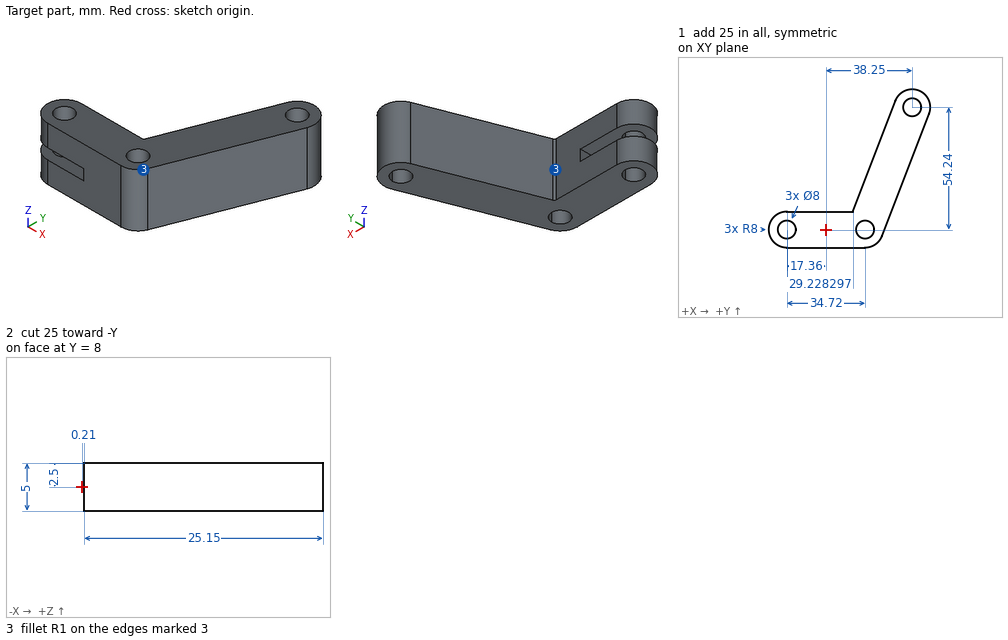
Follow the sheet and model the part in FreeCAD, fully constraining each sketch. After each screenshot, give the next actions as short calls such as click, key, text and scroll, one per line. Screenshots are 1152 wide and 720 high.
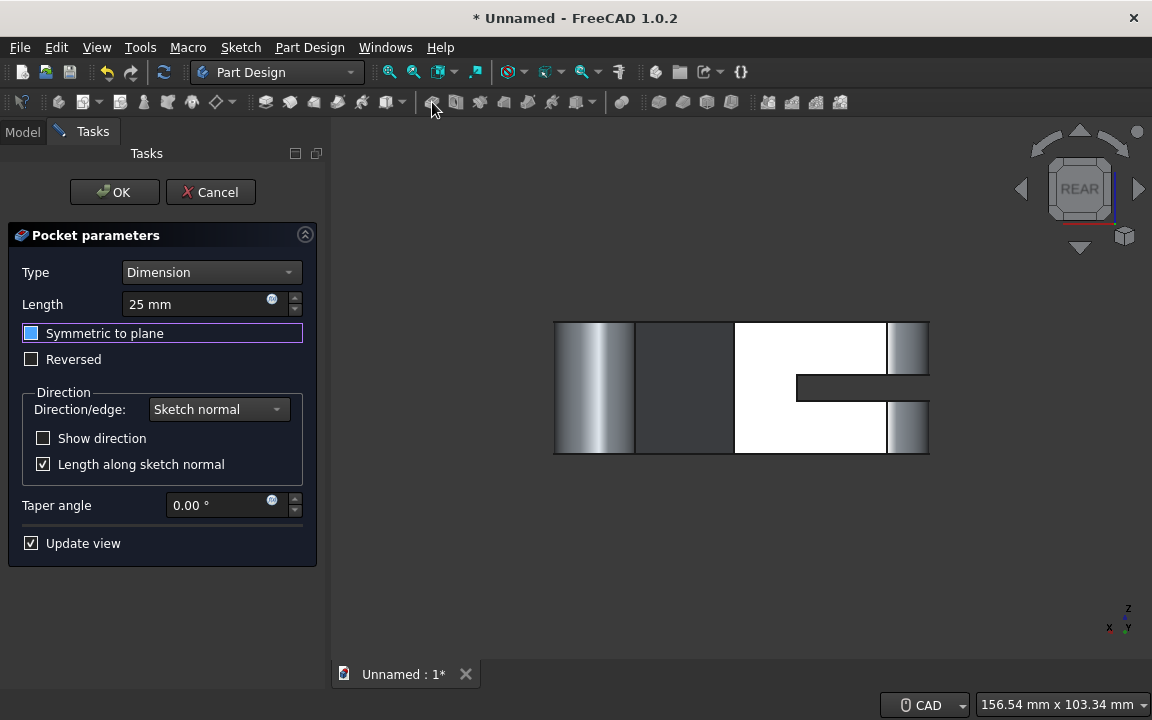
click(115, 192)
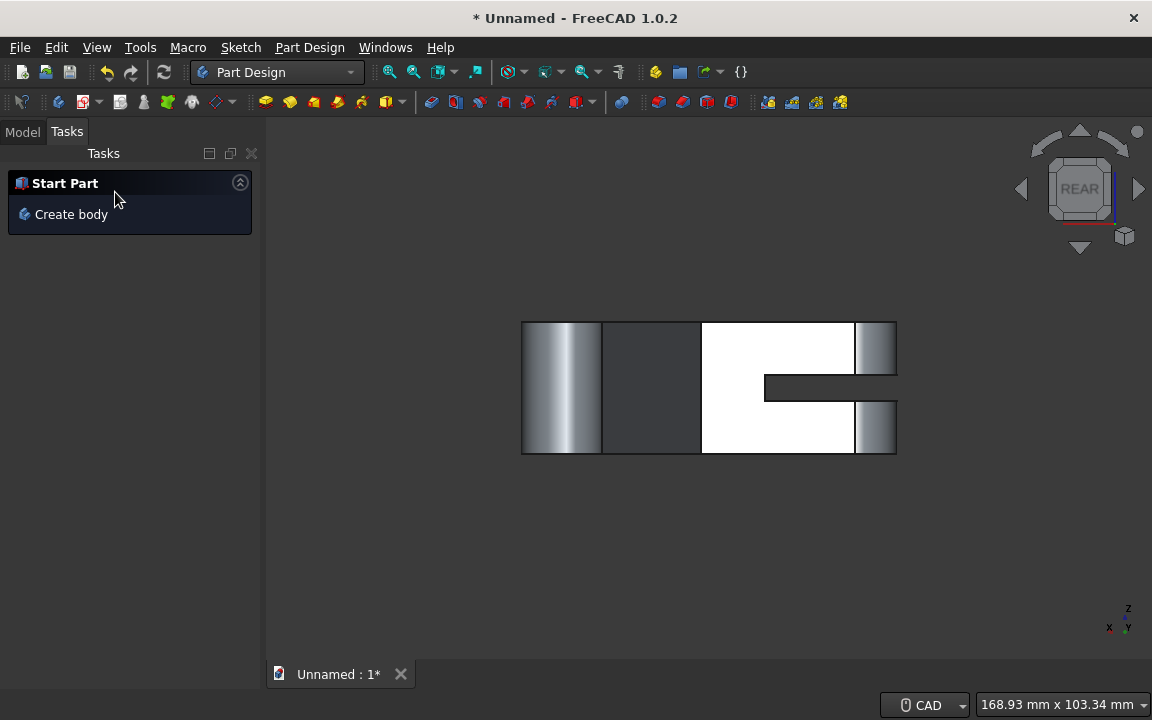
key(v)
key(f)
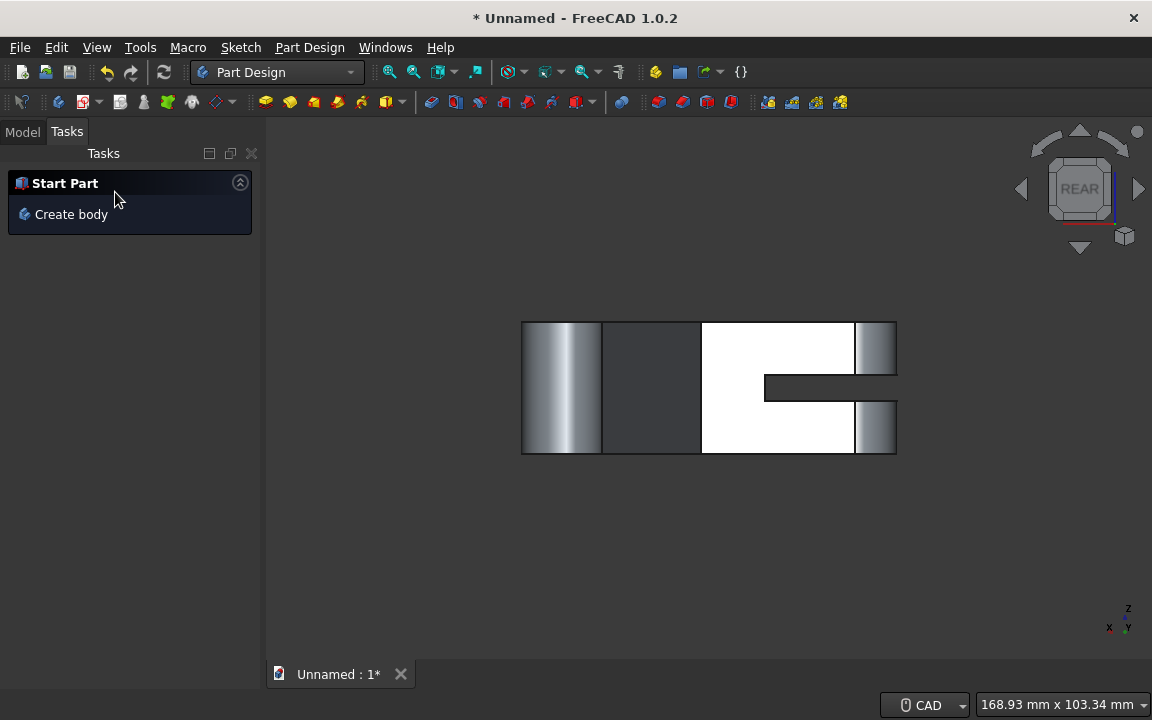
key(0)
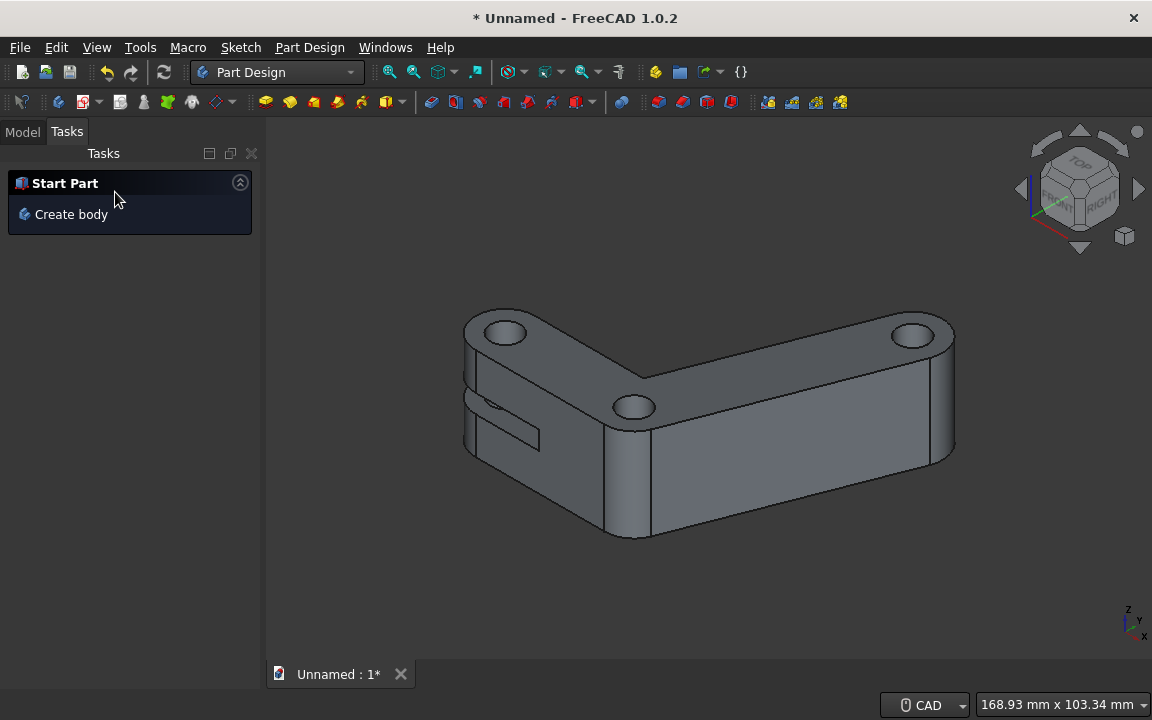
key(2)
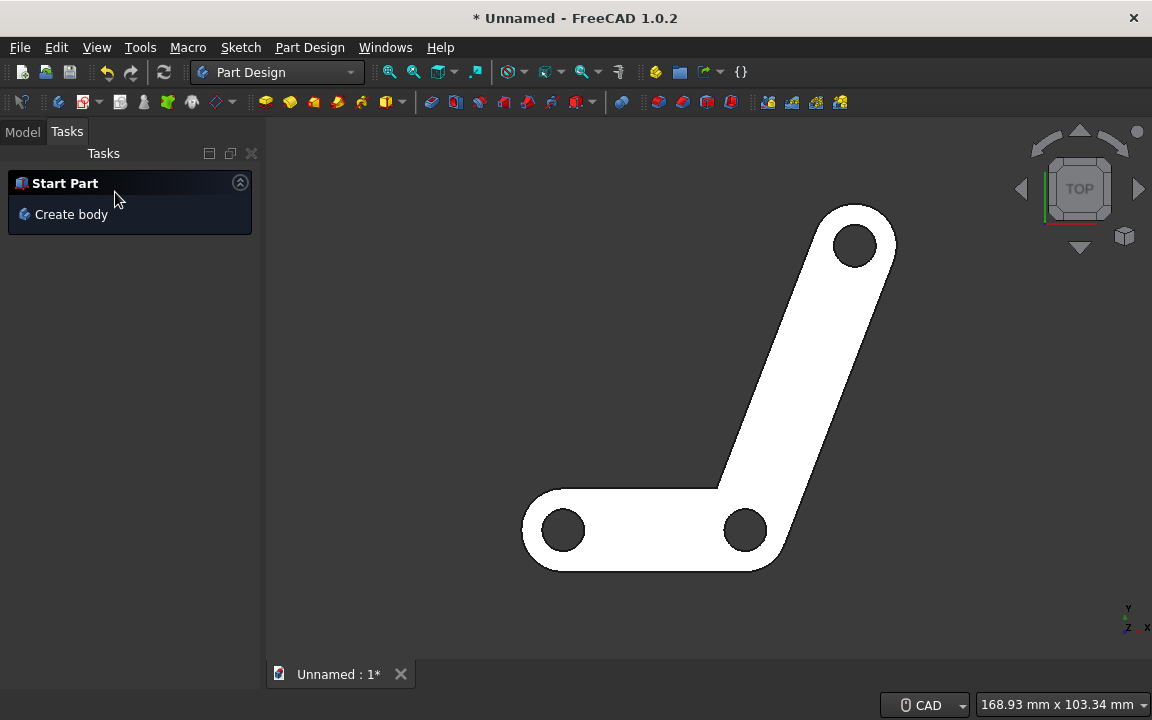
key(1)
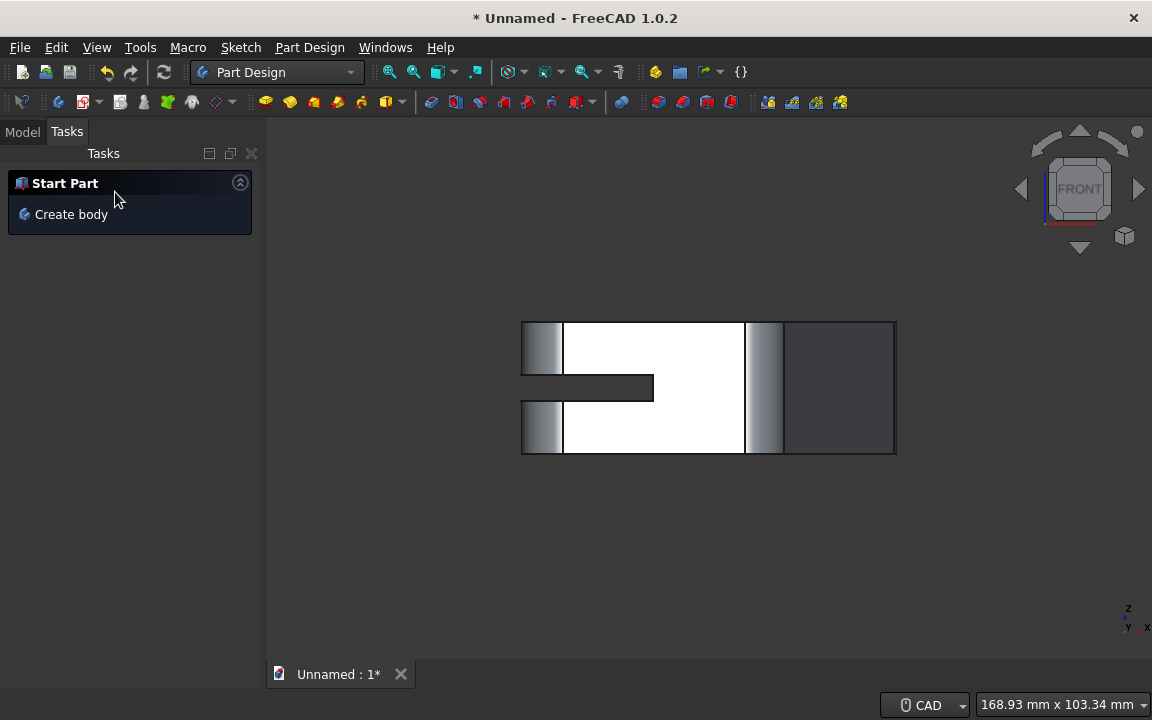
click(390, 72)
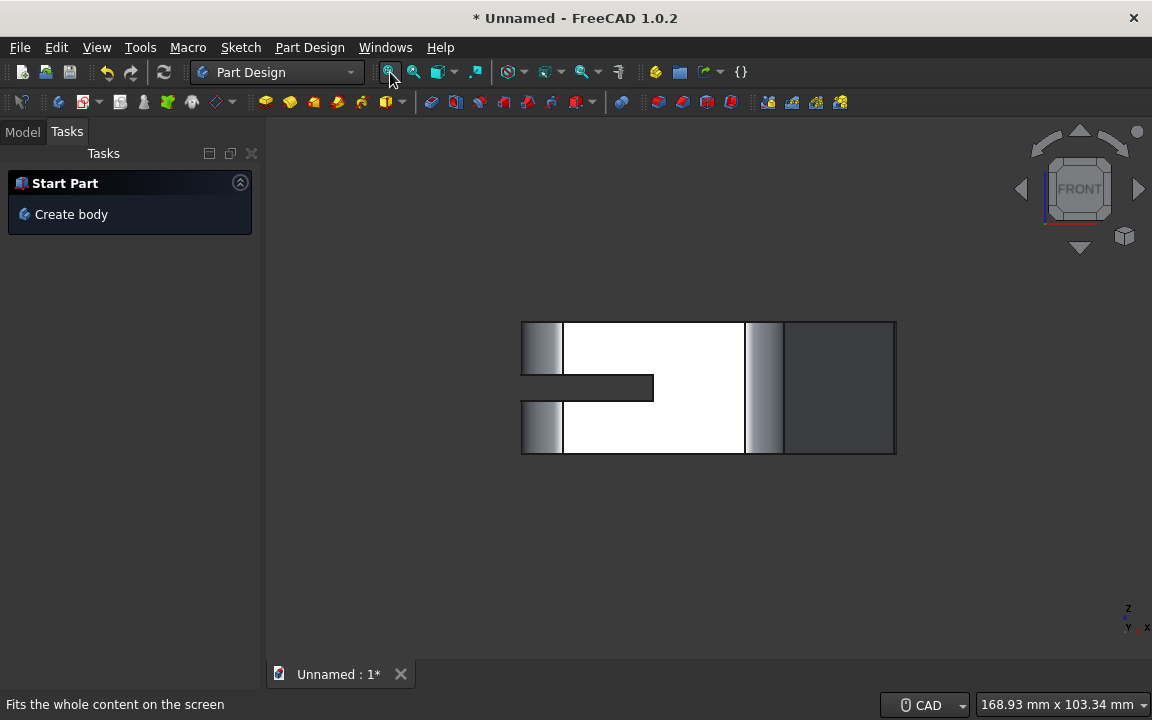
key(3)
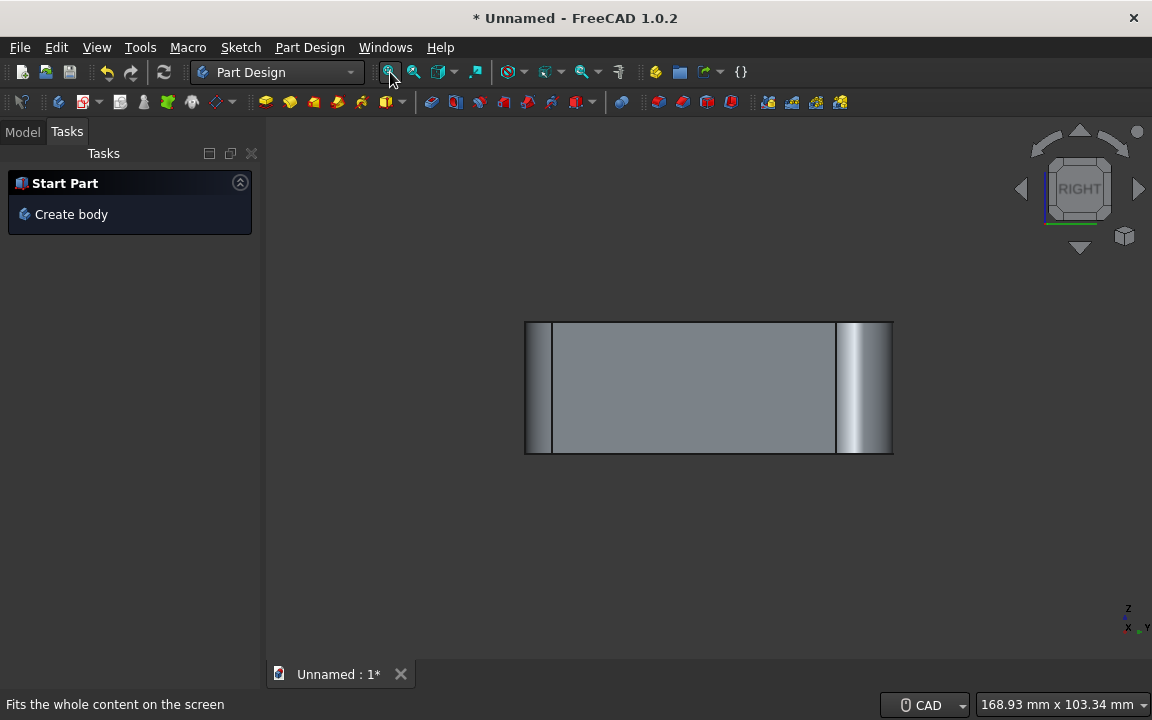
click(390, 72)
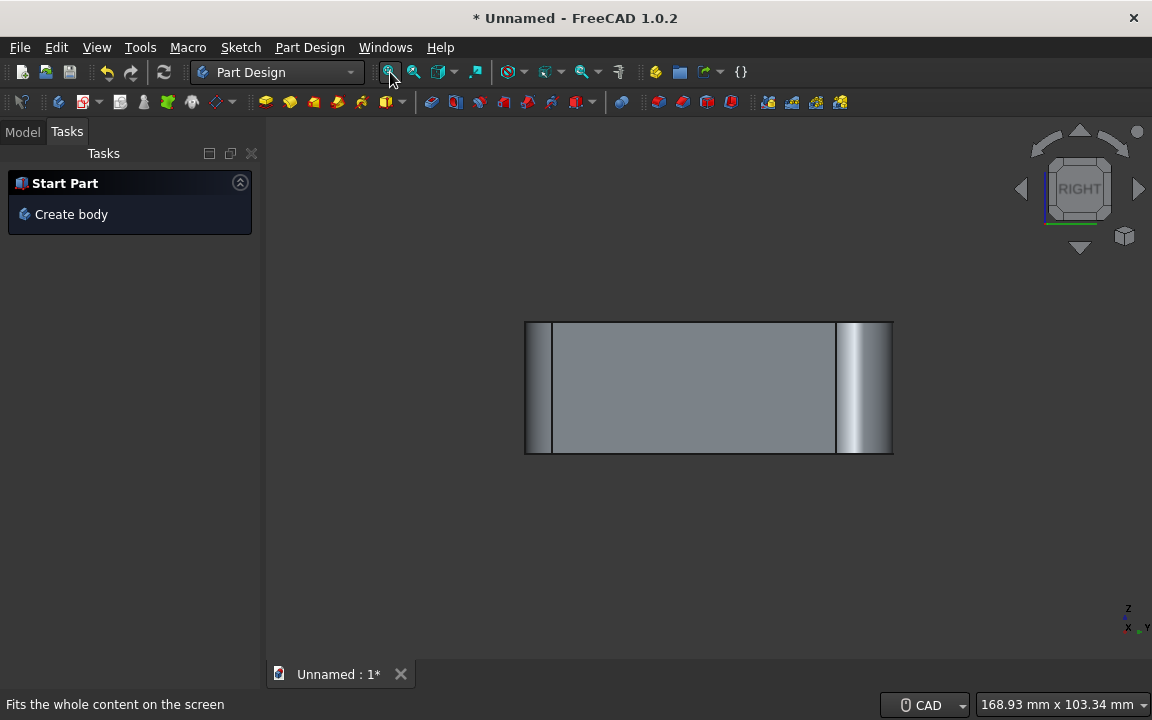
key(5)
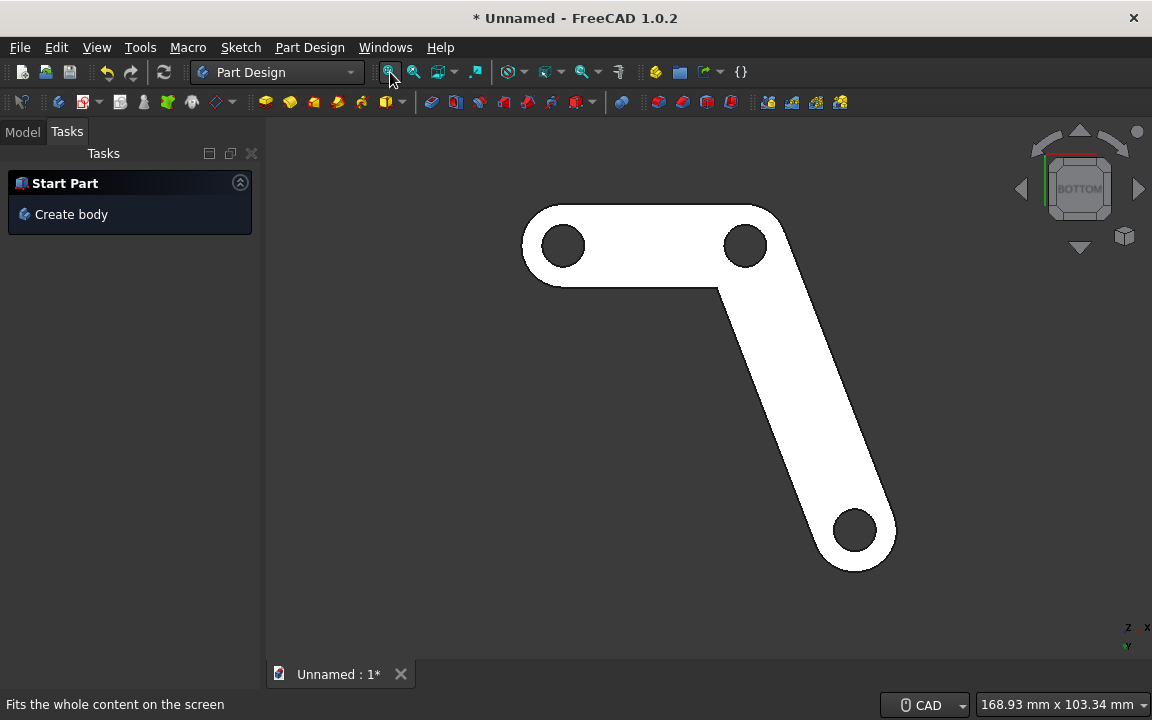
key(4)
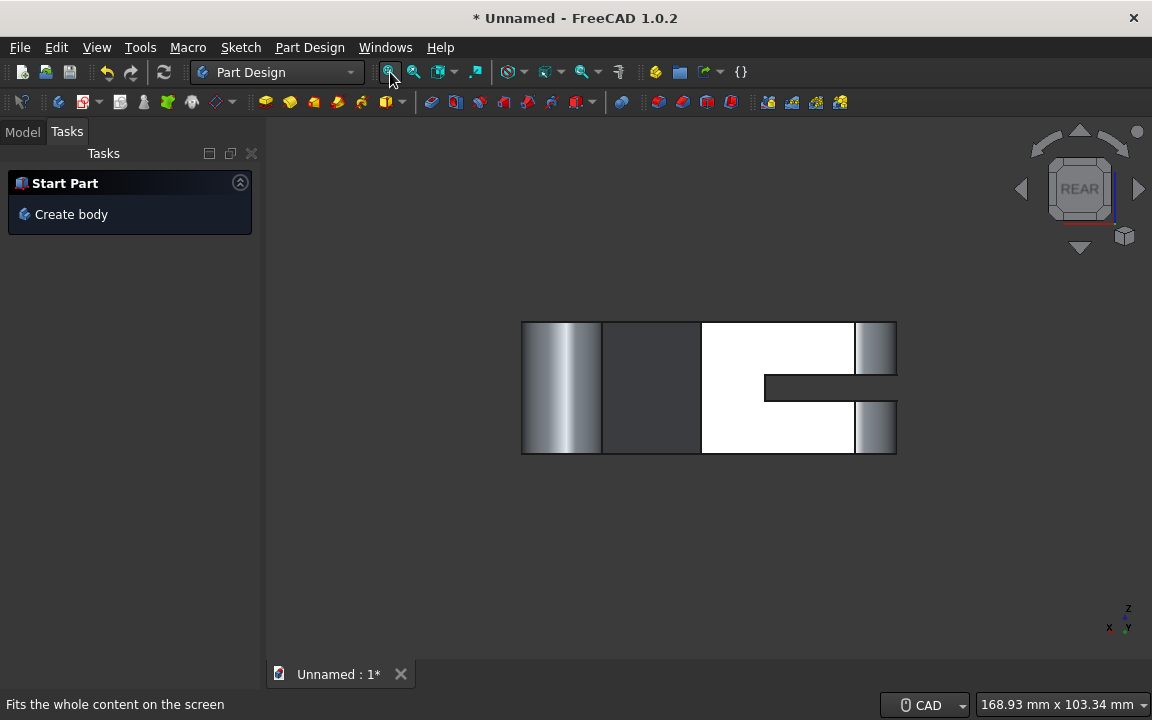
key(v)
key(f)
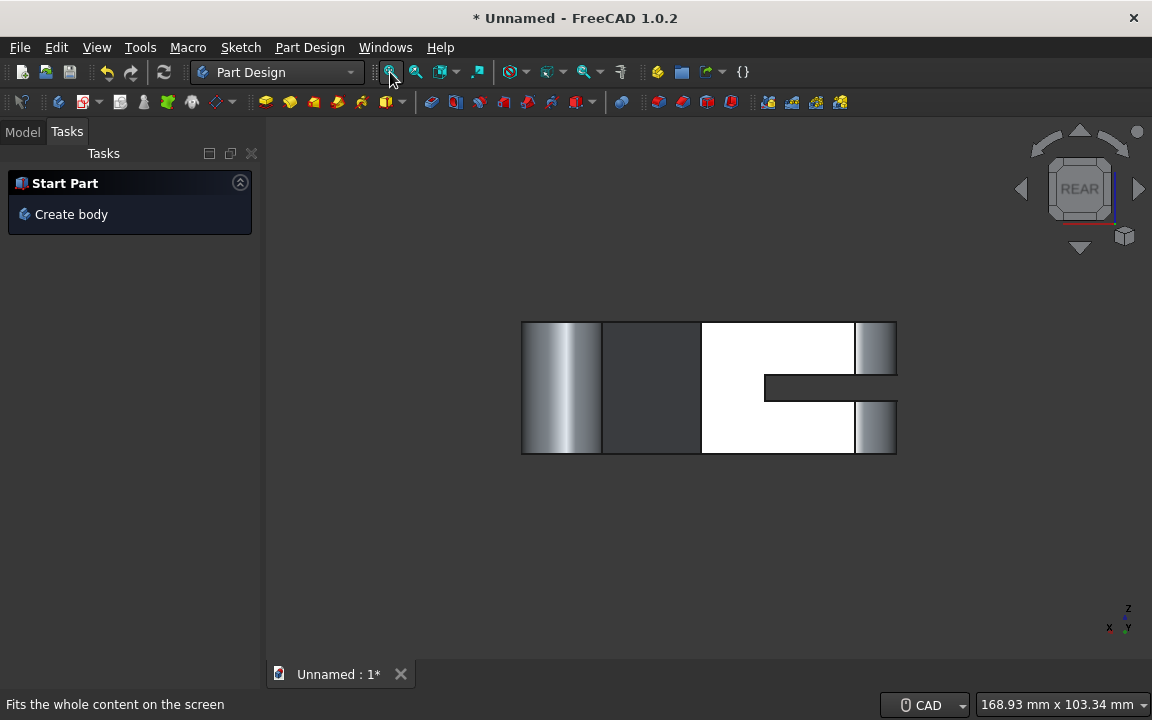
key(6)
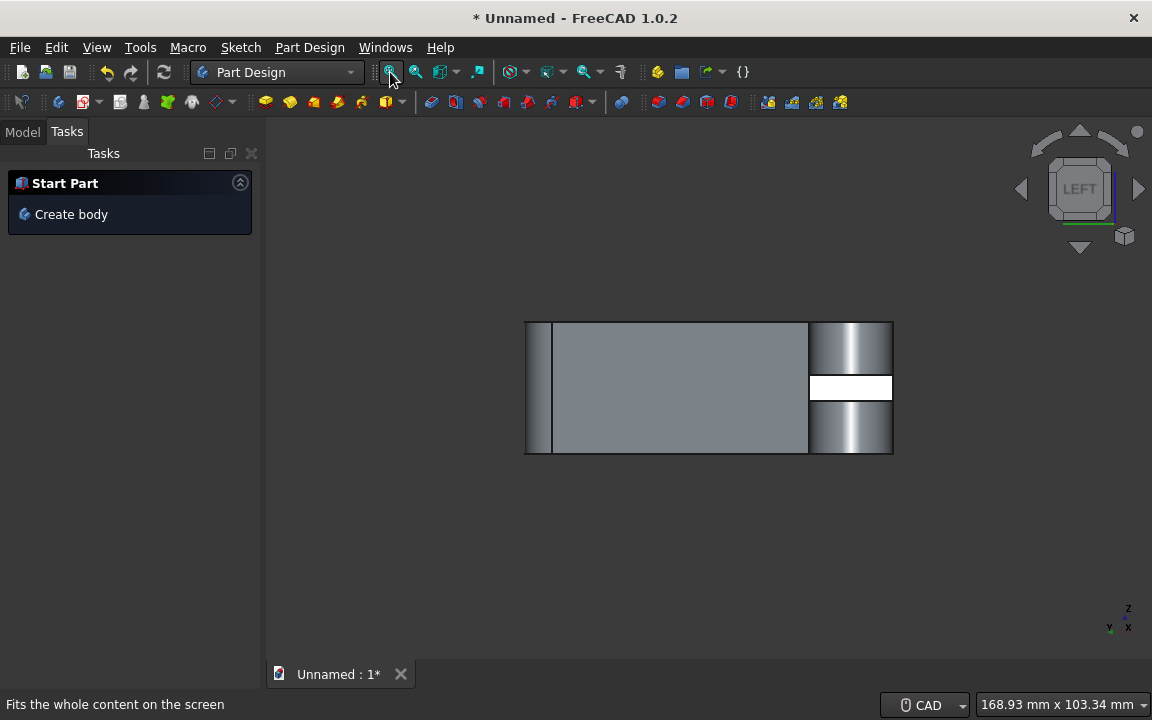
click(392, 72)